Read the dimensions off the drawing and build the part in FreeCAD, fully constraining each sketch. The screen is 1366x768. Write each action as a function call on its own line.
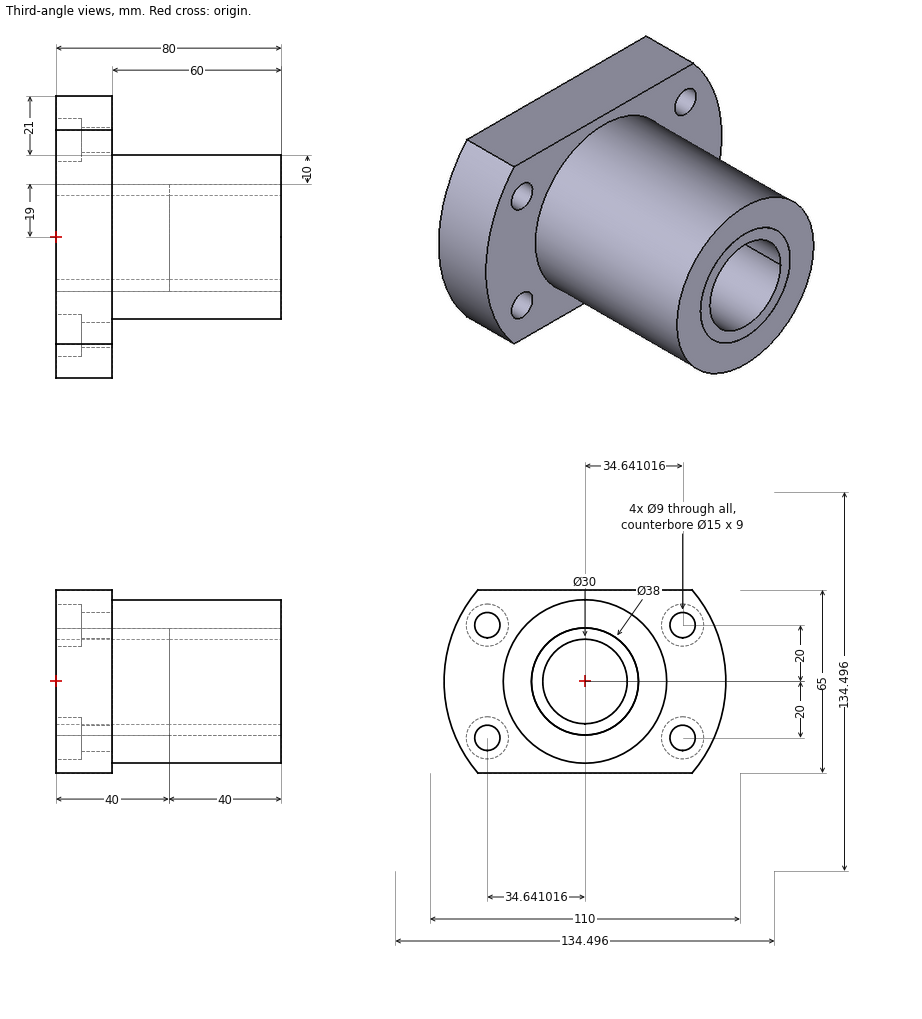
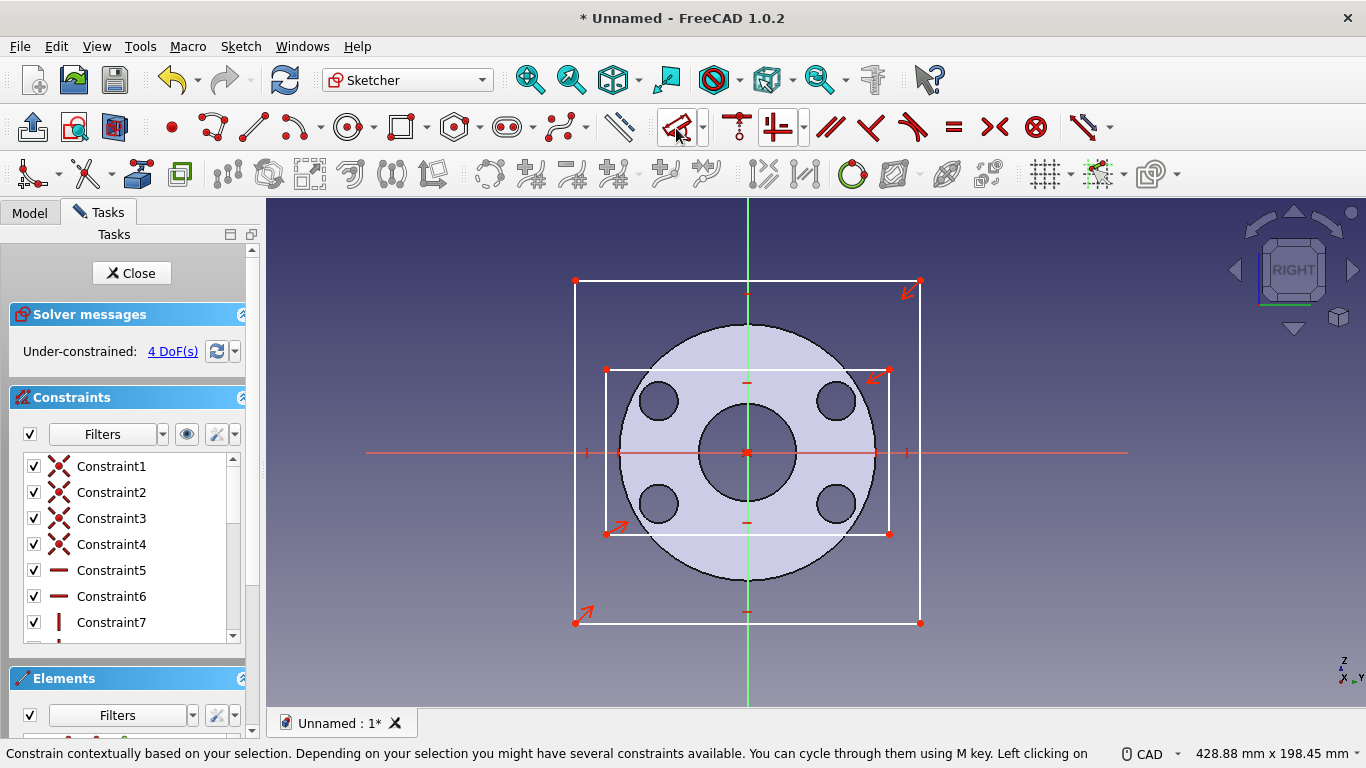
click(889, 485)
click(855, 415)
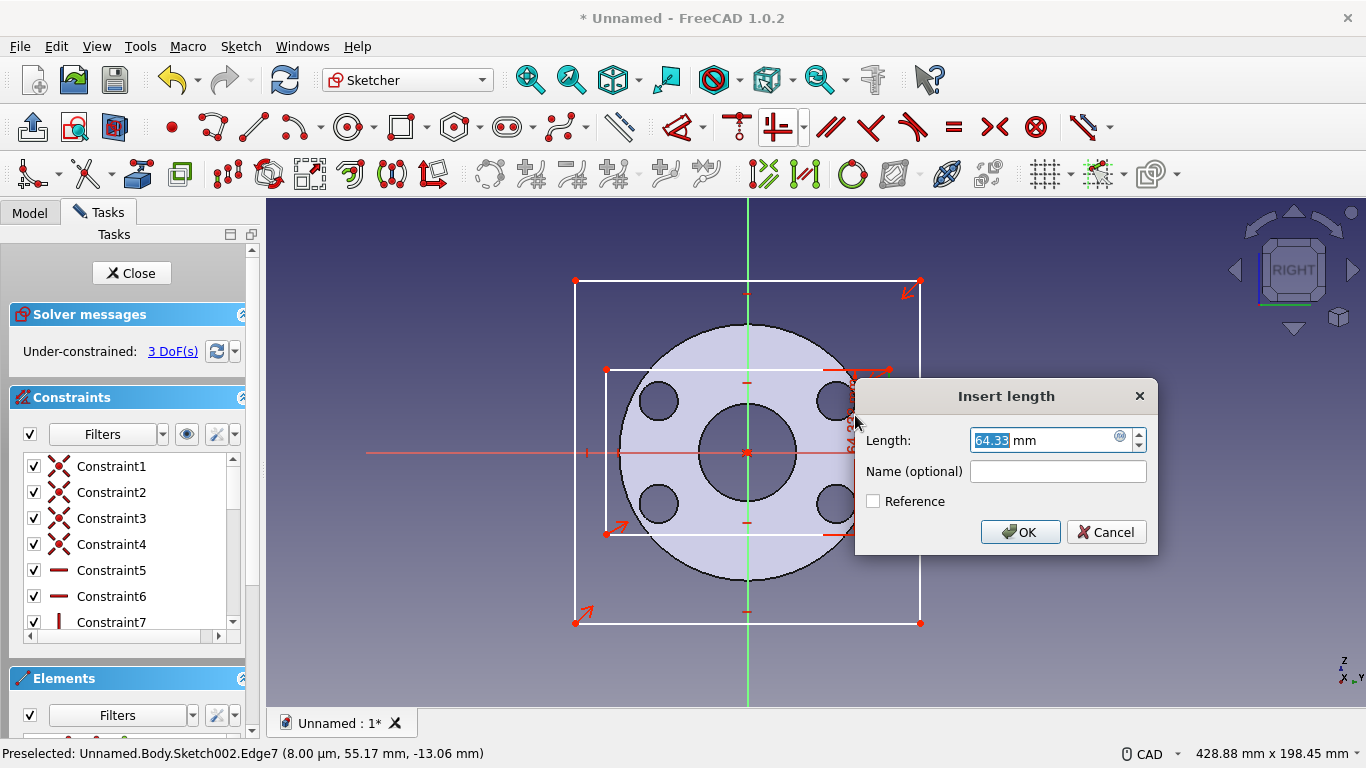
text(65)
key(Return)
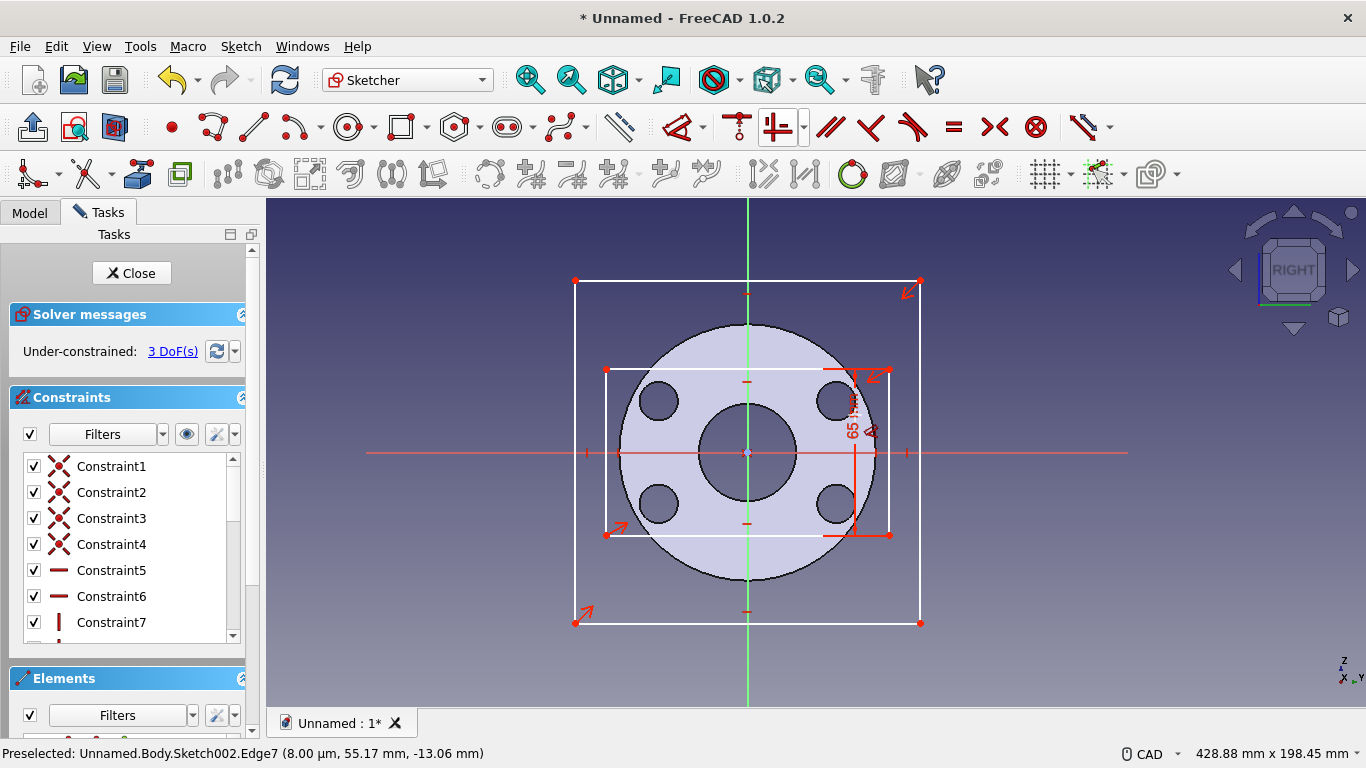
click(691, 536)
click(682, 570)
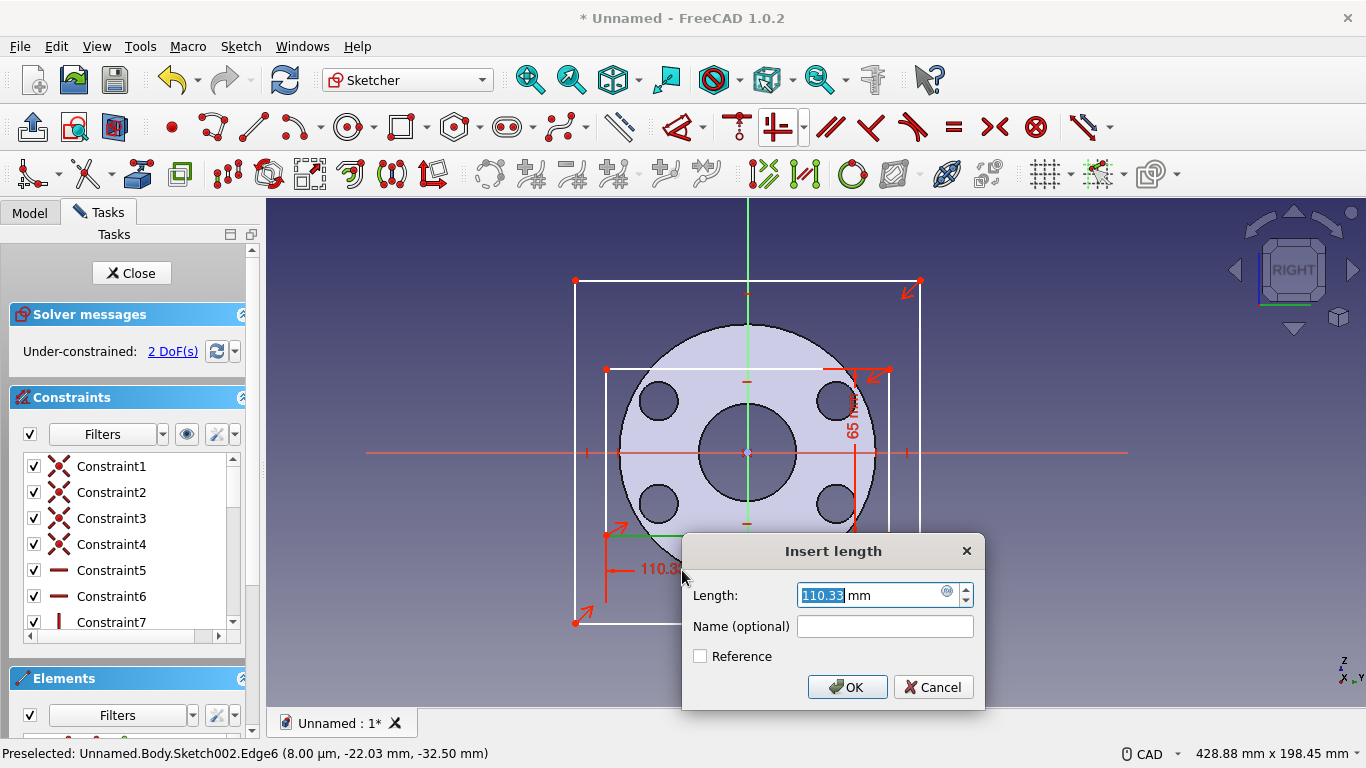
text(110)
key(Return)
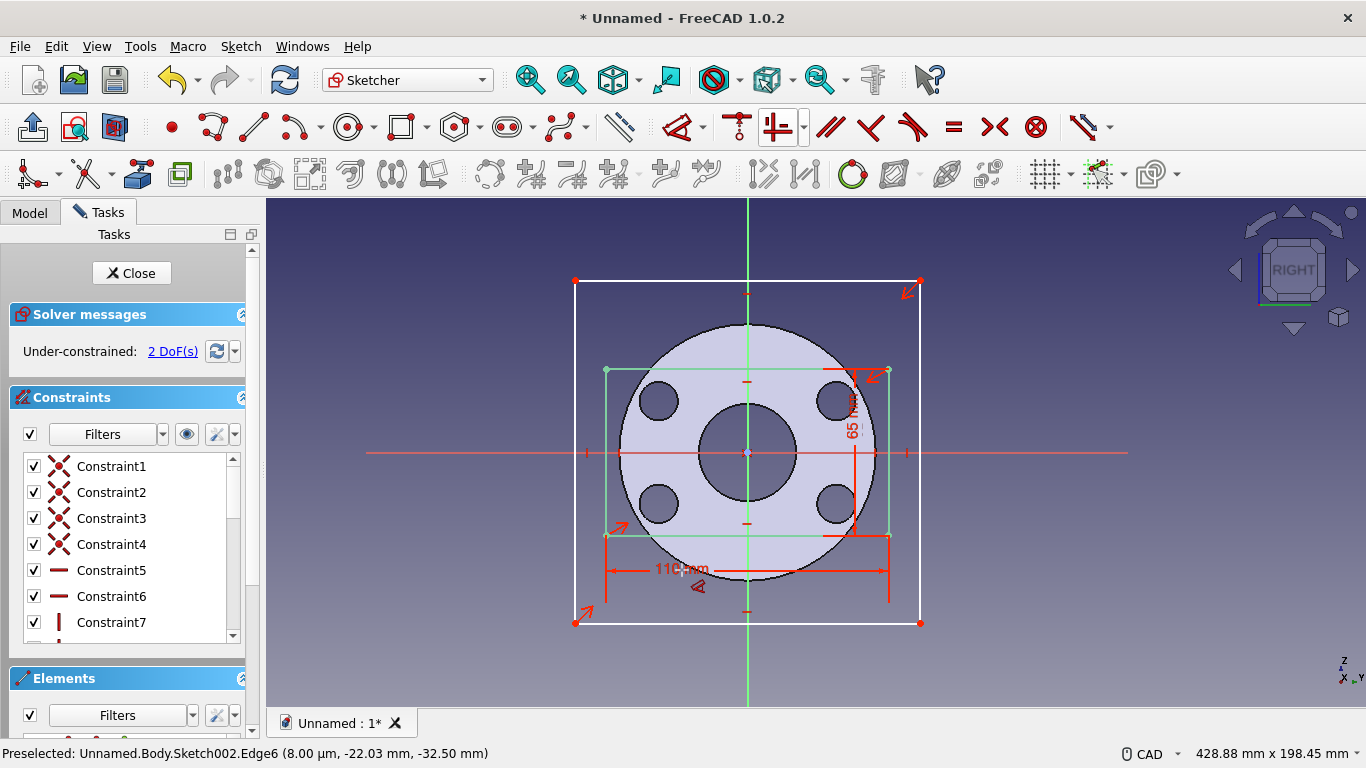
click(679, 624)
click(668, 658)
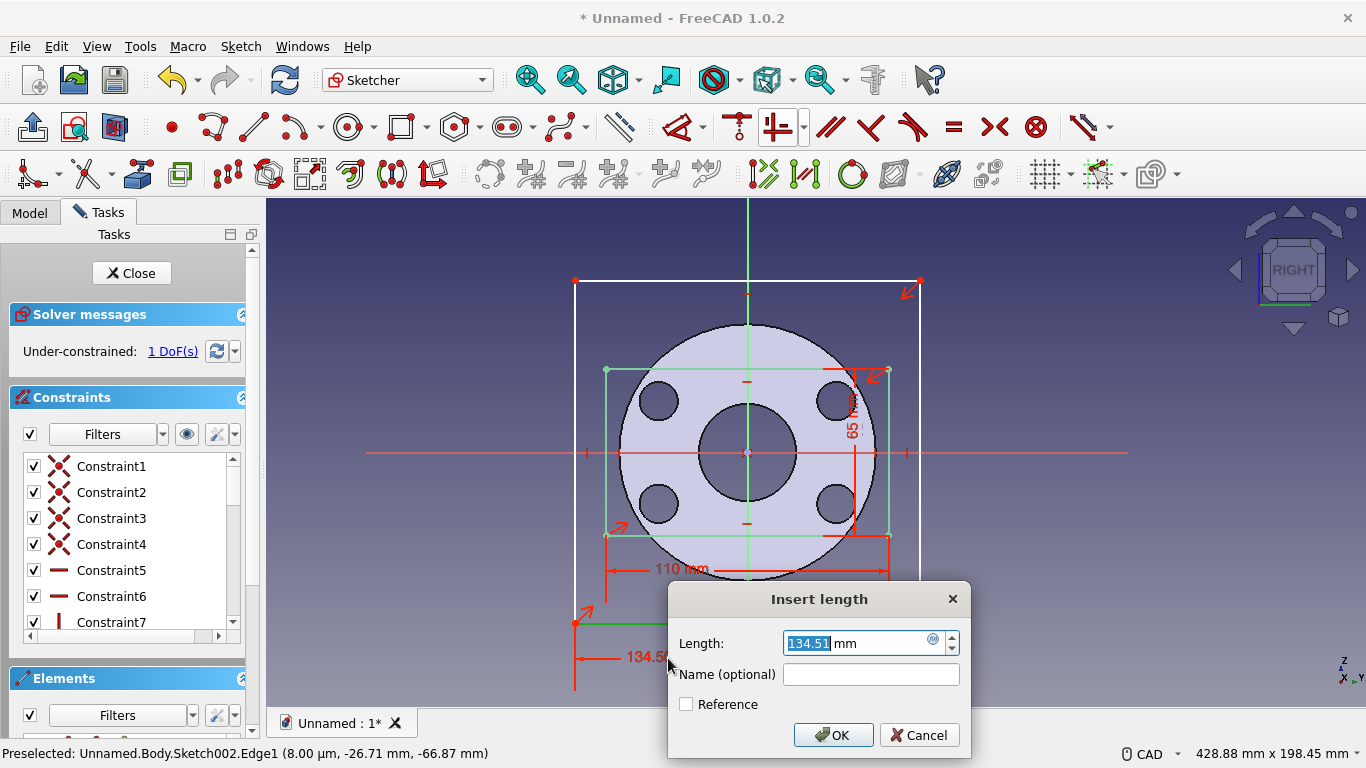
text(134.496)
key(Return)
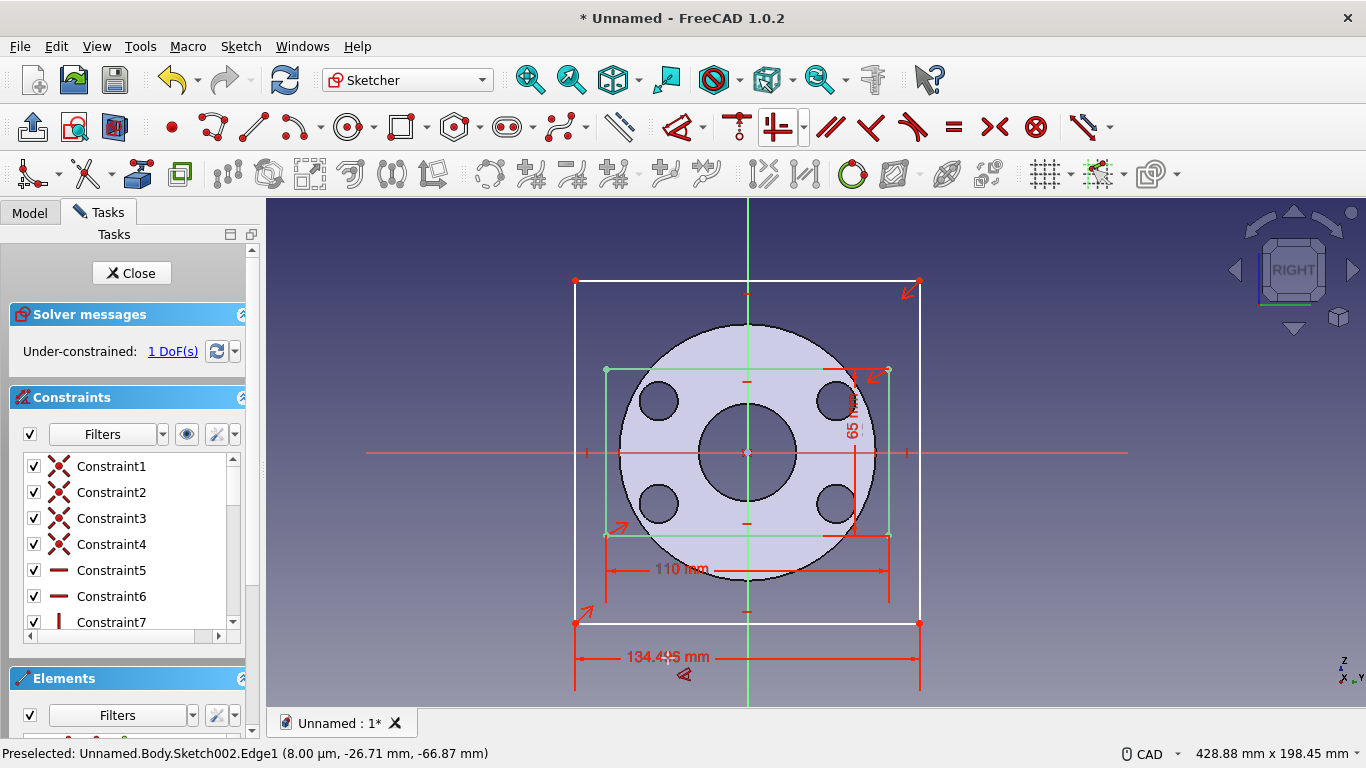
click(920, 521)
click(954, 374)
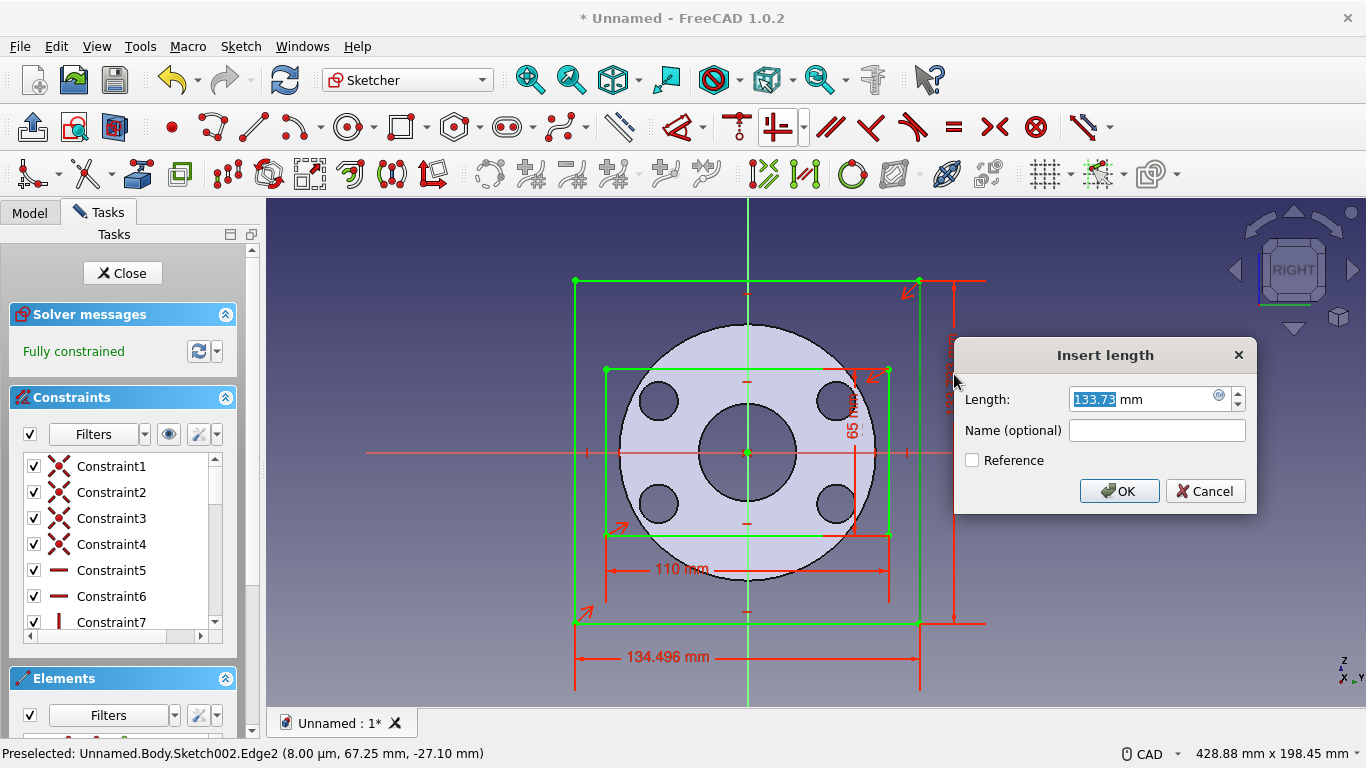
text(134.496)
key(Return)
key(Escape)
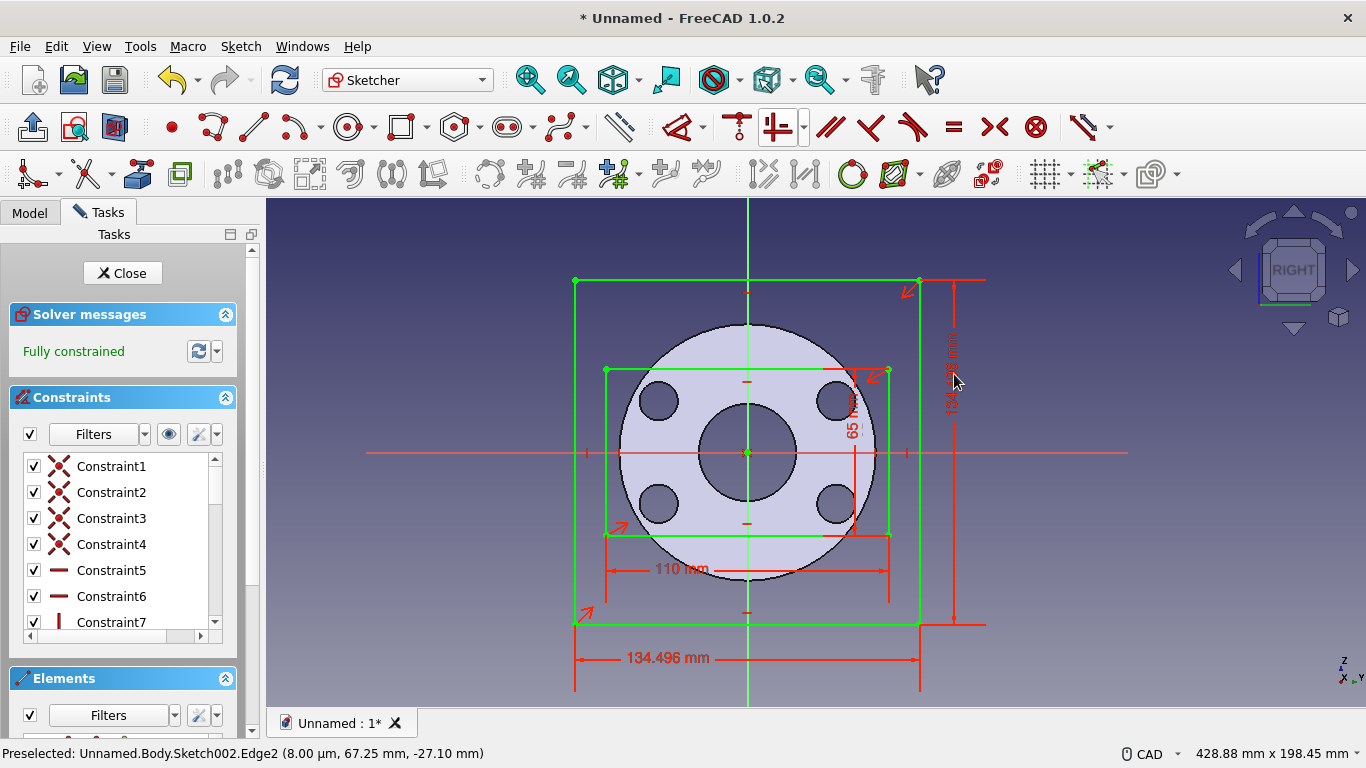
click(123, 273)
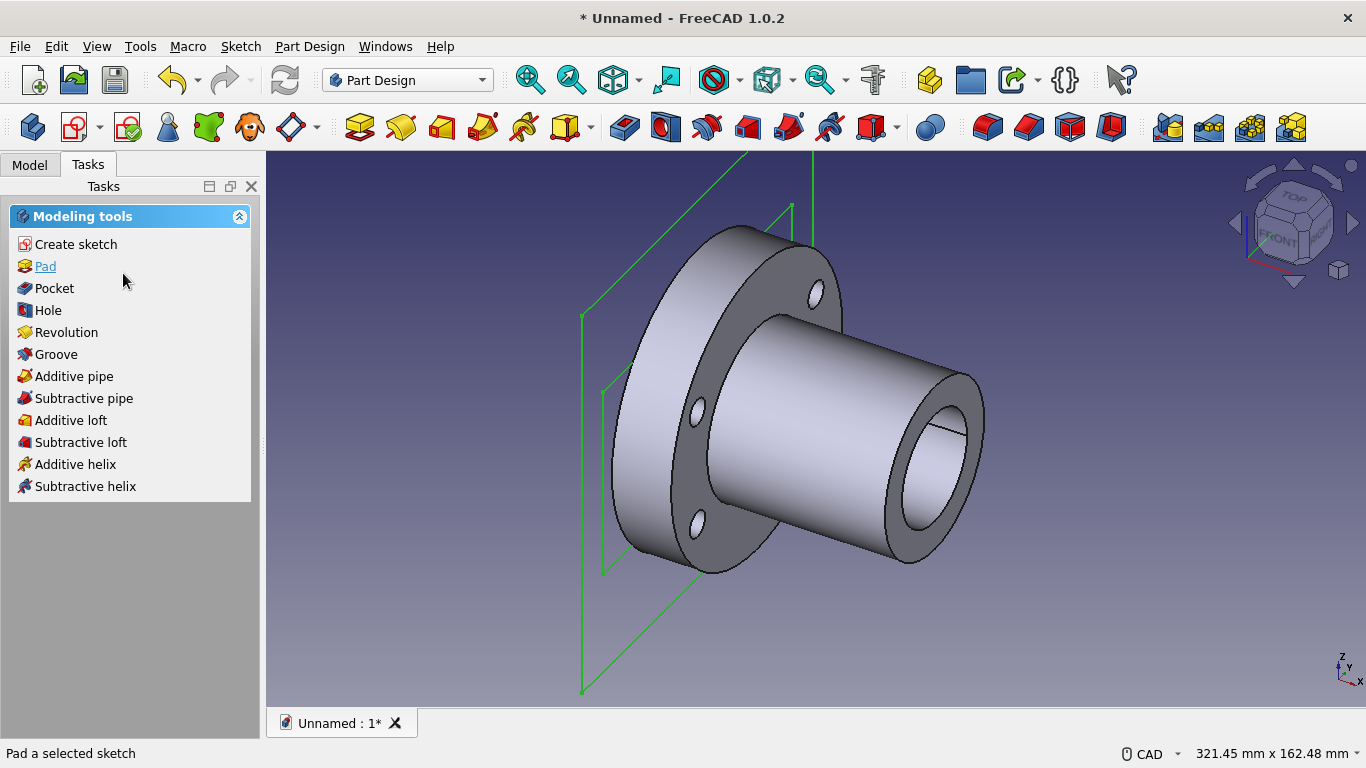
click(625, 128)